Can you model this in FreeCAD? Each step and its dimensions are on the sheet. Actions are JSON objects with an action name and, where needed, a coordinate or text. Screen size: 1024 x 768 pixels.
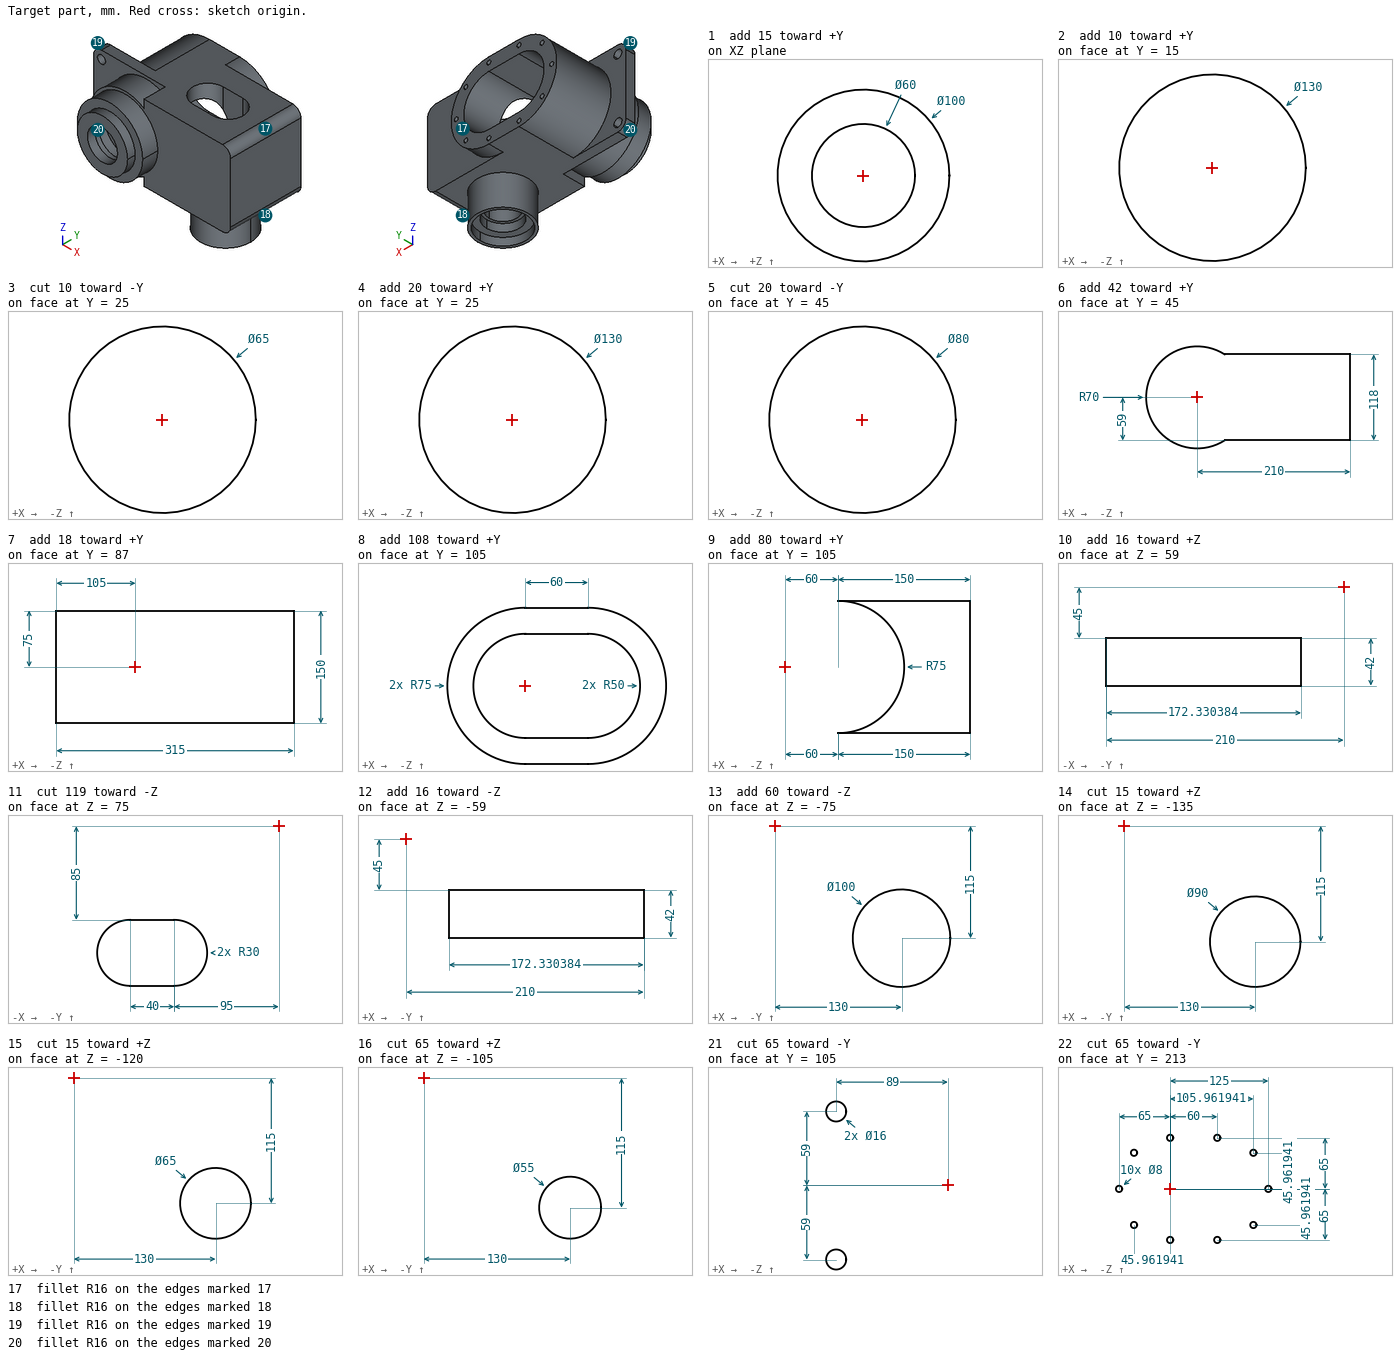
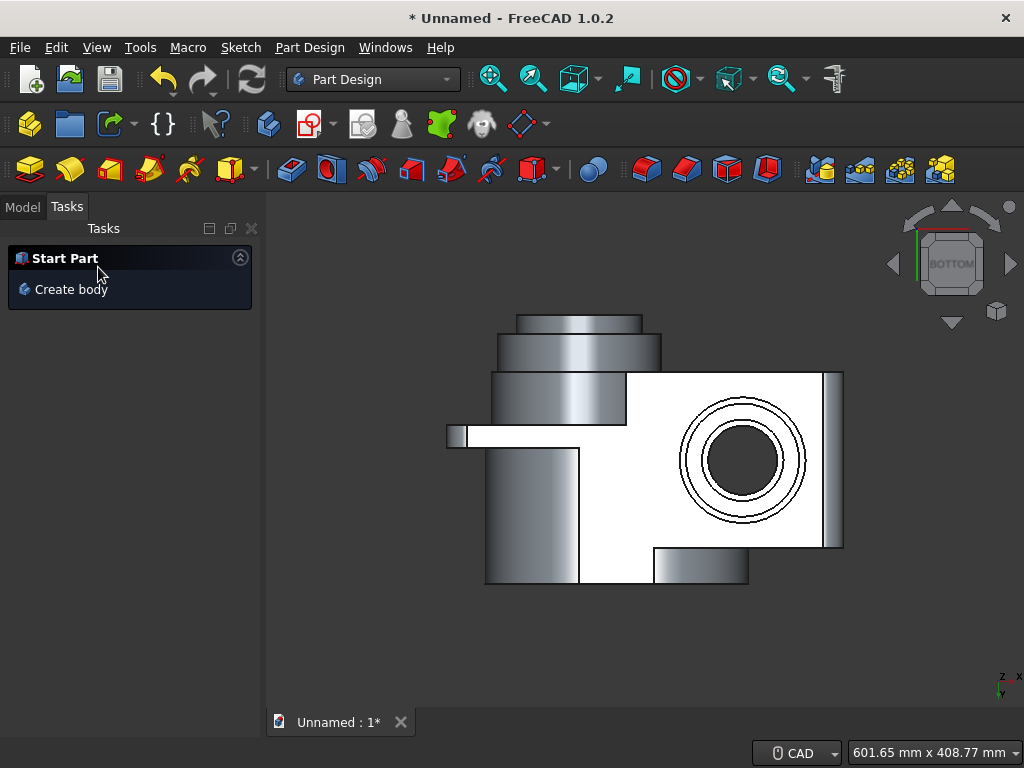
{"action": "key", "text": "4"}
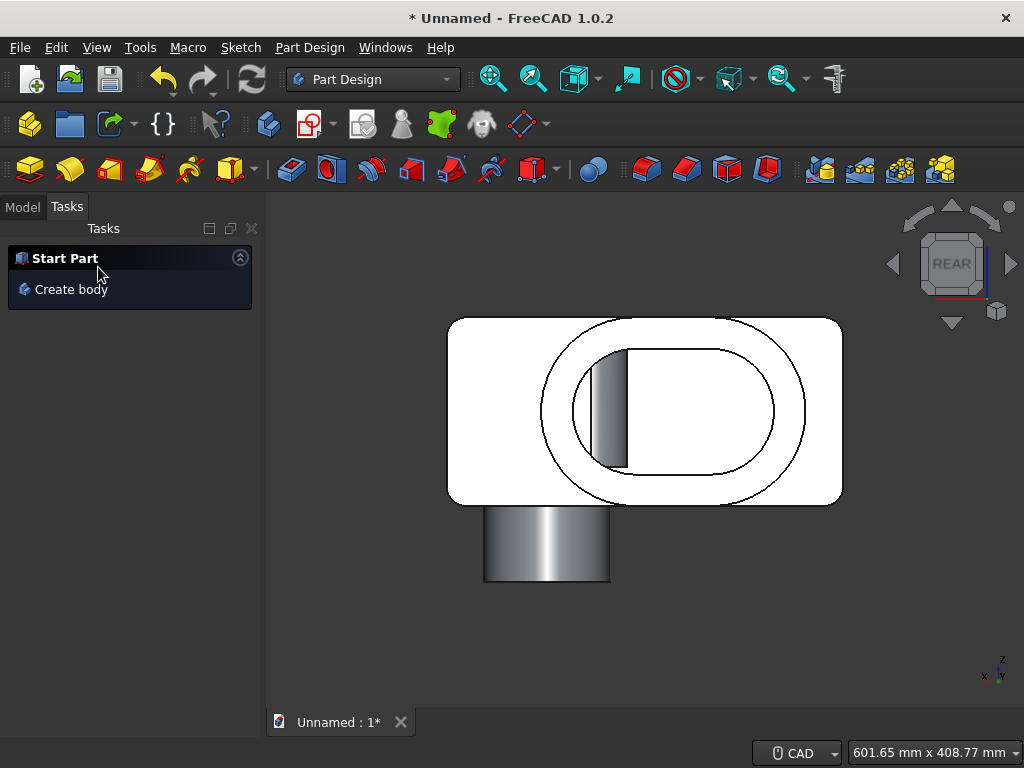
{"action": "left_click", "coordinate": [690, 411]}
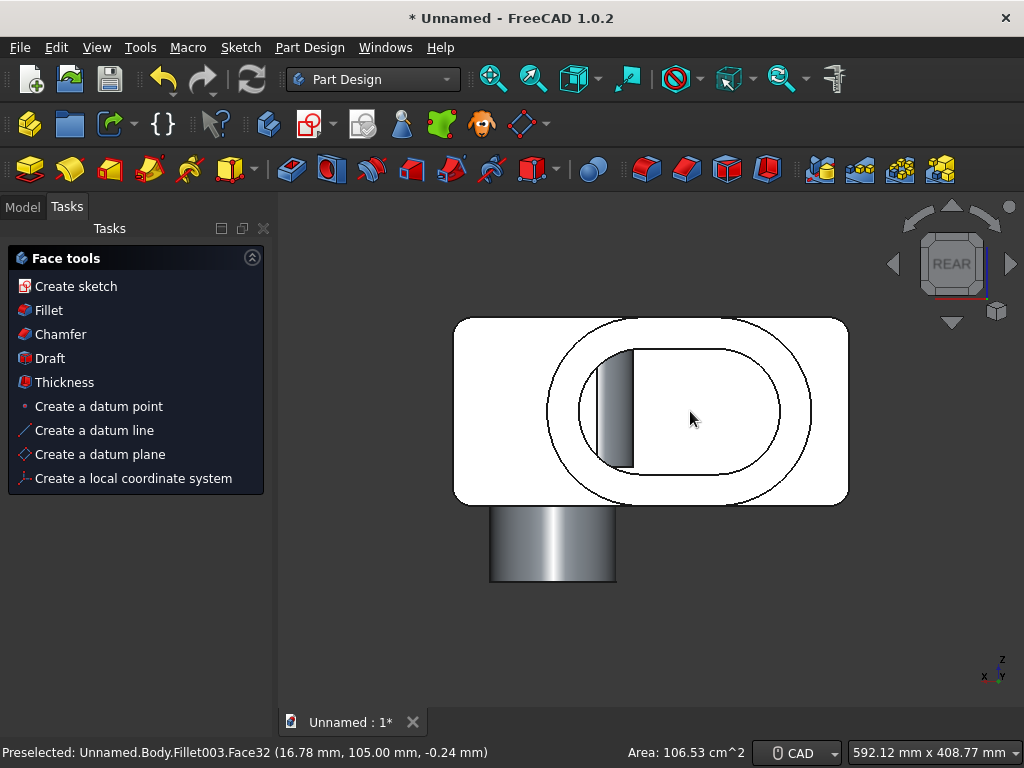
{"action": "left_click", "coordinate": [310, 124]}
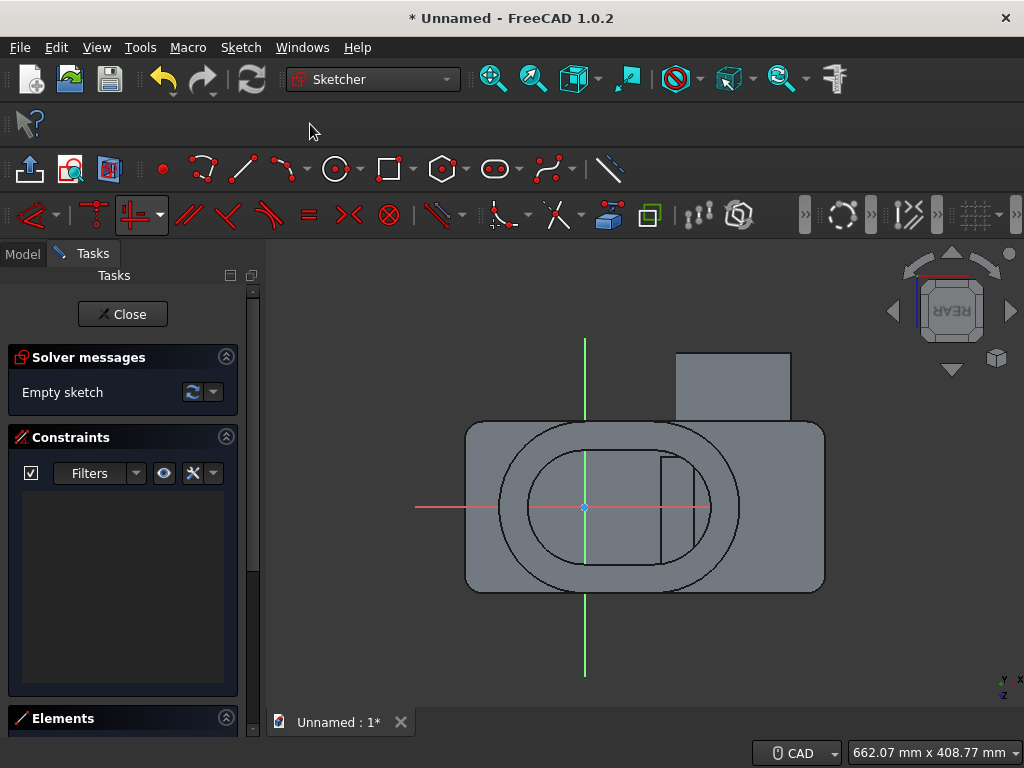
{"action": "left_click", "coordinate": [110, 170]}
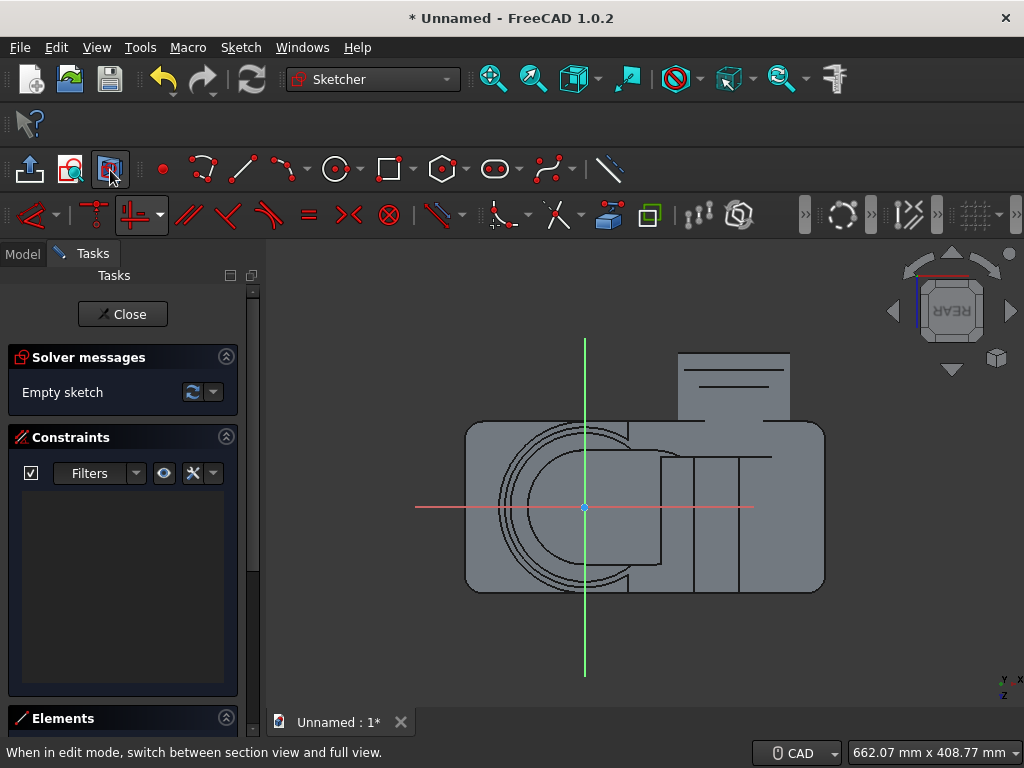
{"action": "scroll", "coordinate": [472, 549], "scroll_direction": "up", "scroll_amount": 3}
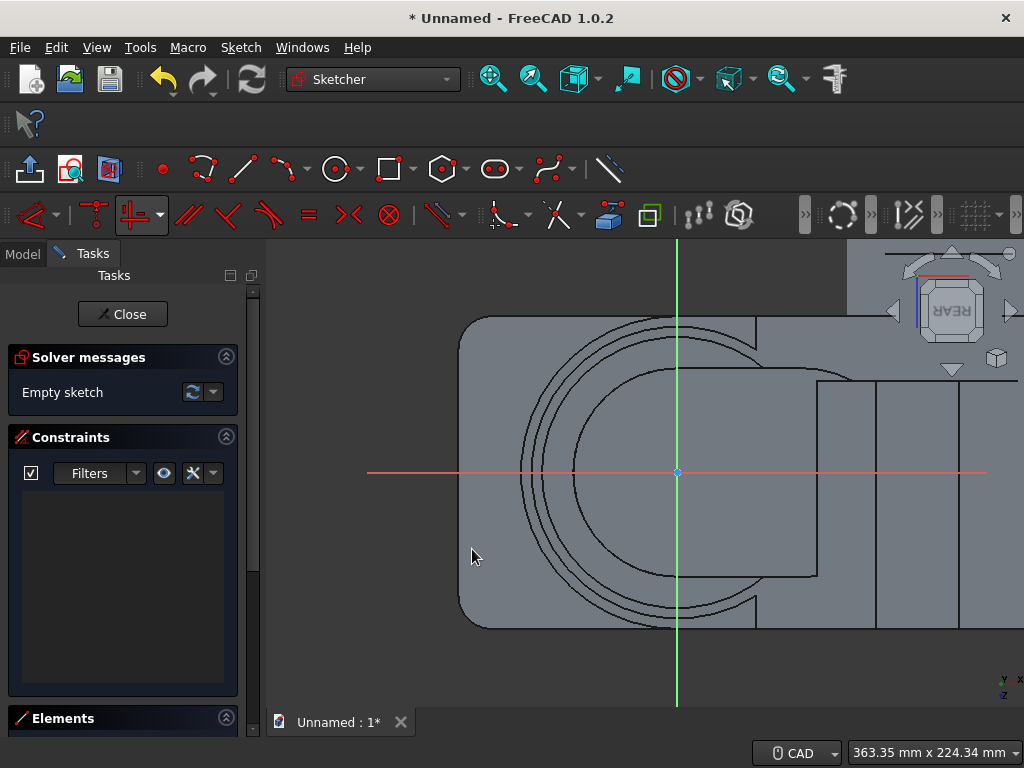
{"action": "left_click", "coordinate": [336, 170]}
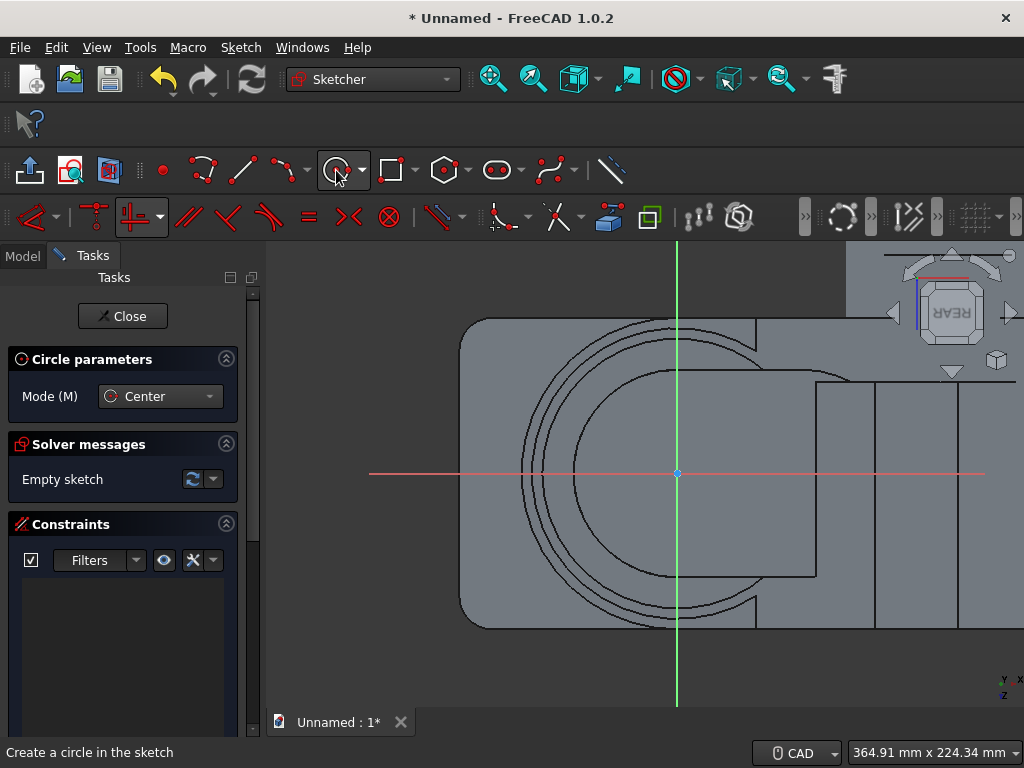
{"action": "scroll", "coordinate": [492, 351], "scroll_direction": "up", "scroll_amount": 2}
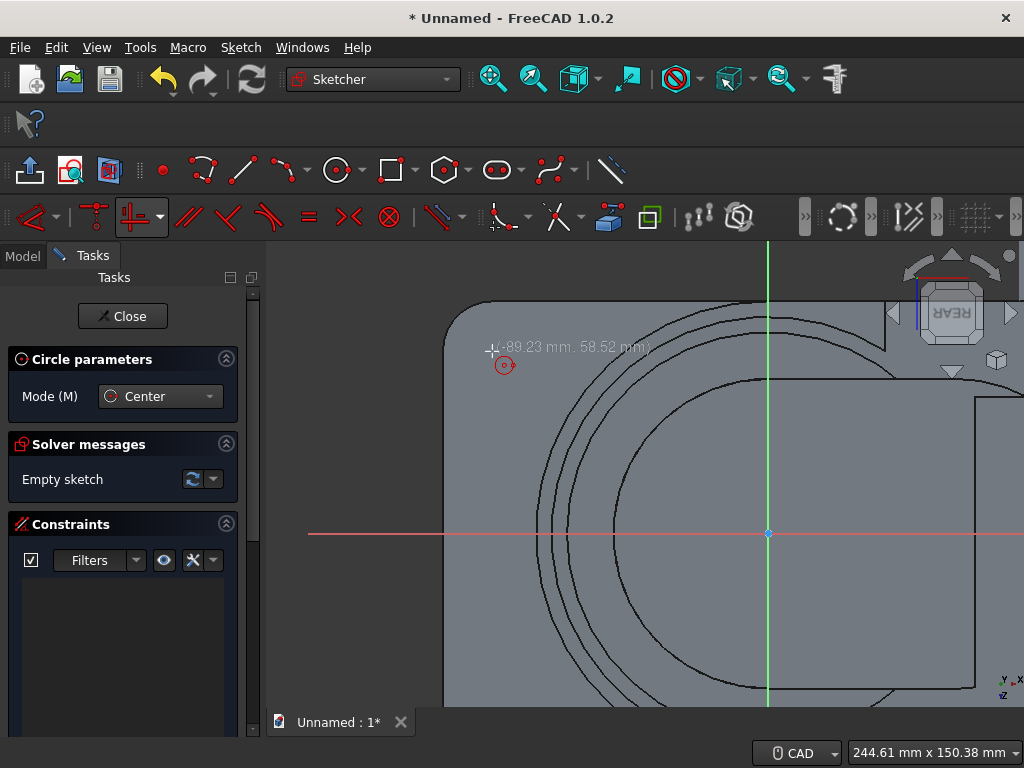
{"action": "left_click", "coordinate": [493, 351]}
{"action": "mouse_move", "coordinate": [510, 333]}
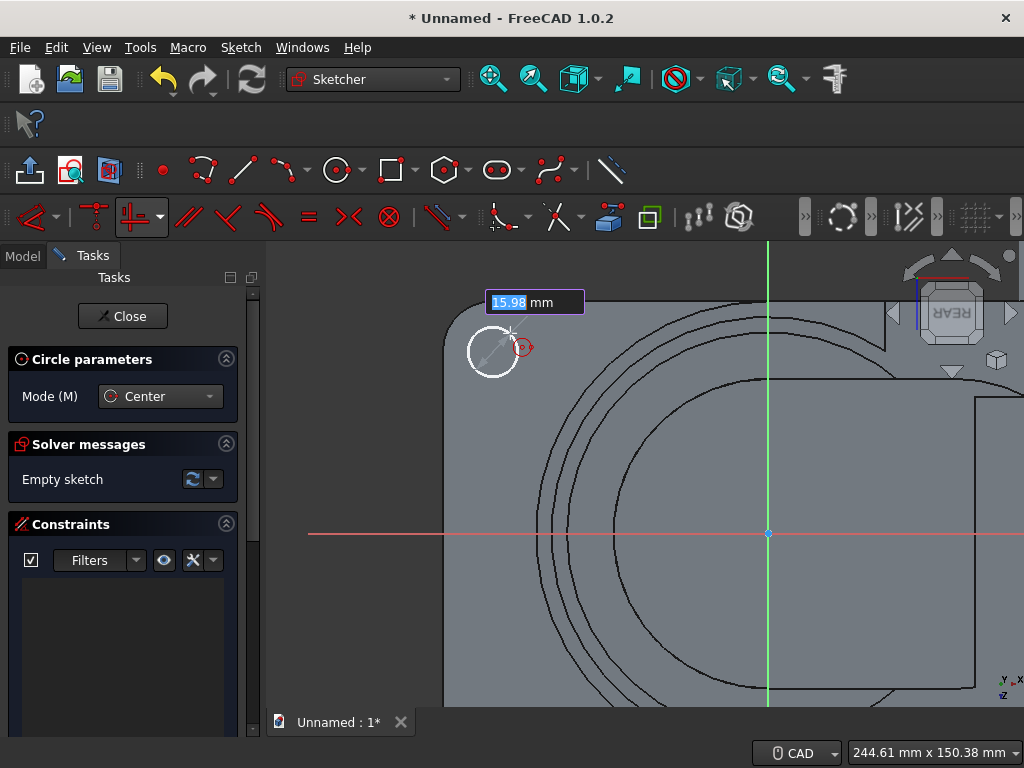
{"action": "type", "text": "16"}
{"action": "key", "text": "Return"}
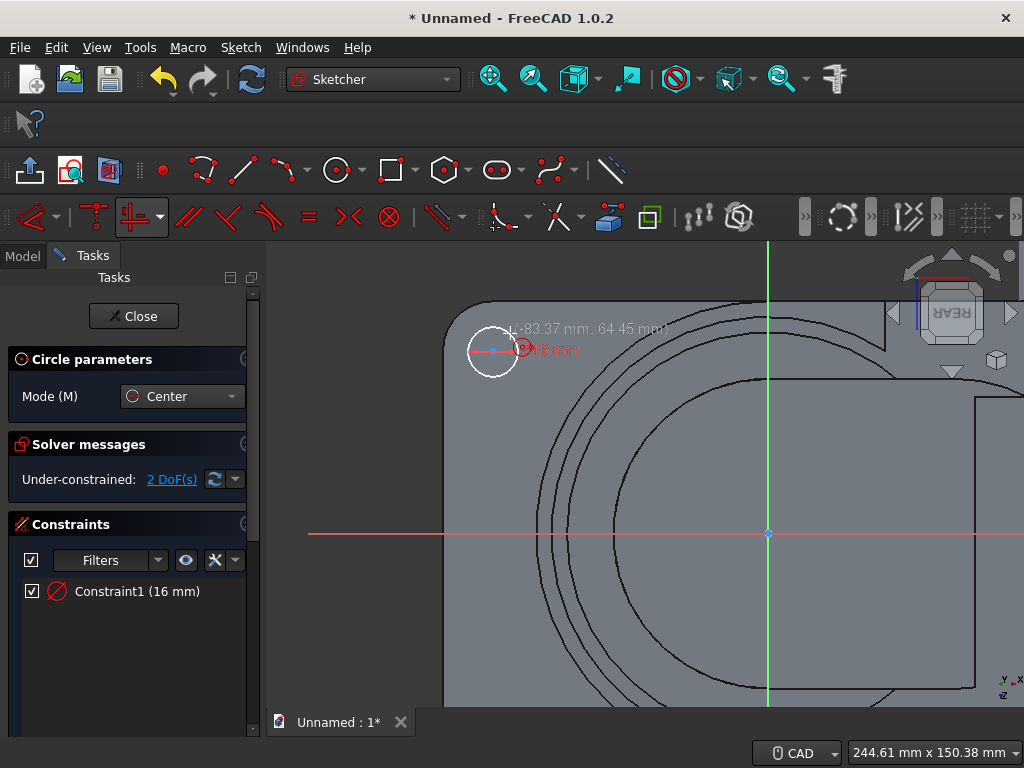
{"action": "scroll", "coordinate": [492, 353], "scroll_direction": "down", "scroll_amount": 2}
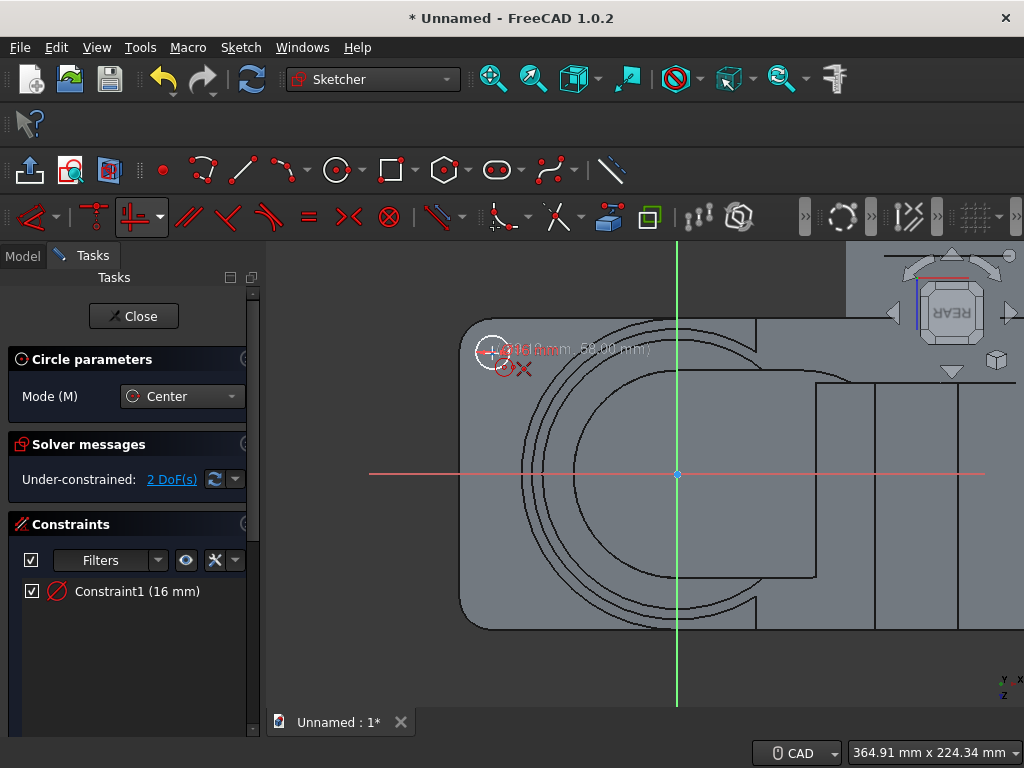
{"action": "scroll", "coordinate": [492, 597], "scroll_direction": "up", "scroll_amount": 2}